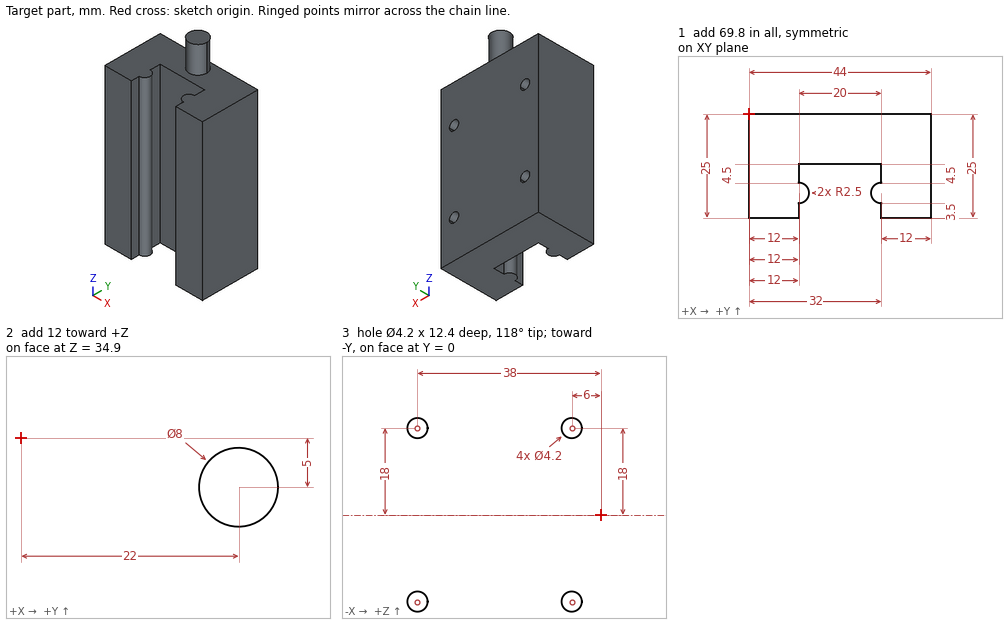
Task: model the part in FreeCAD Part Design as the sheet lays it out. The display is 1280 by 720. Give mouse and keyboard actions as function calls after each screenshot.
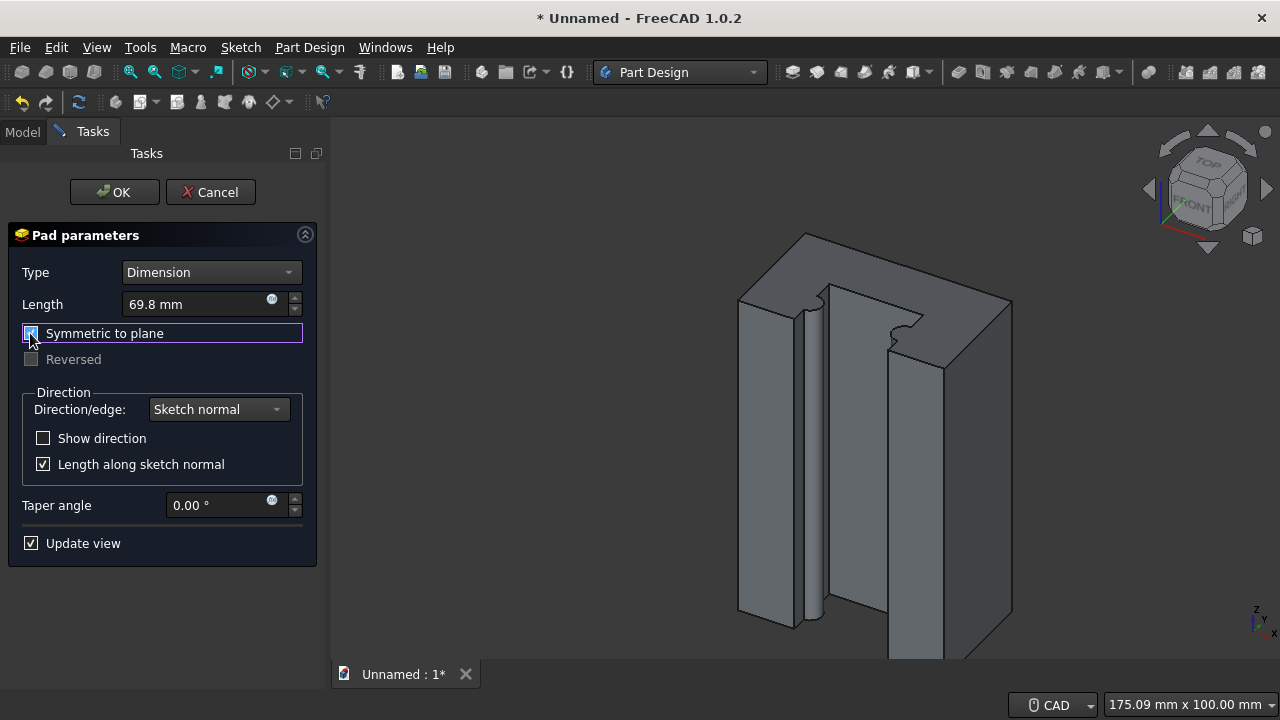
click(115, 192)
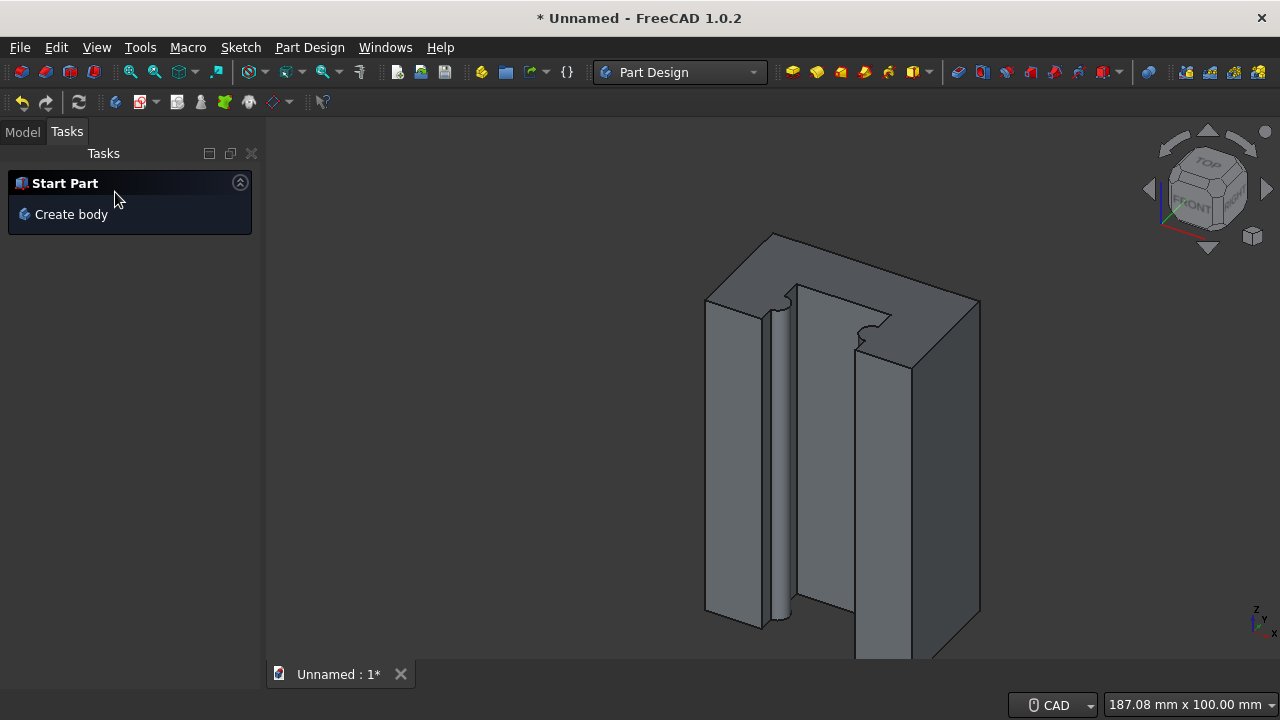
click(132, 72)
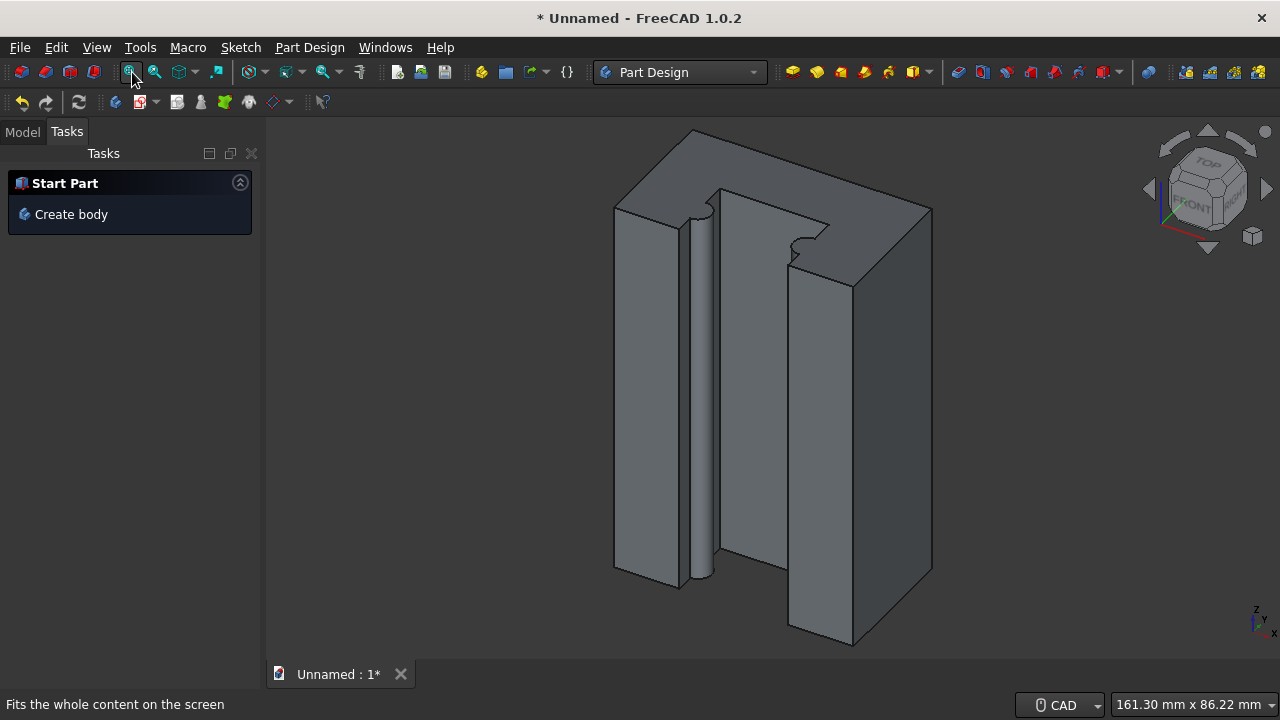
click(864, 208)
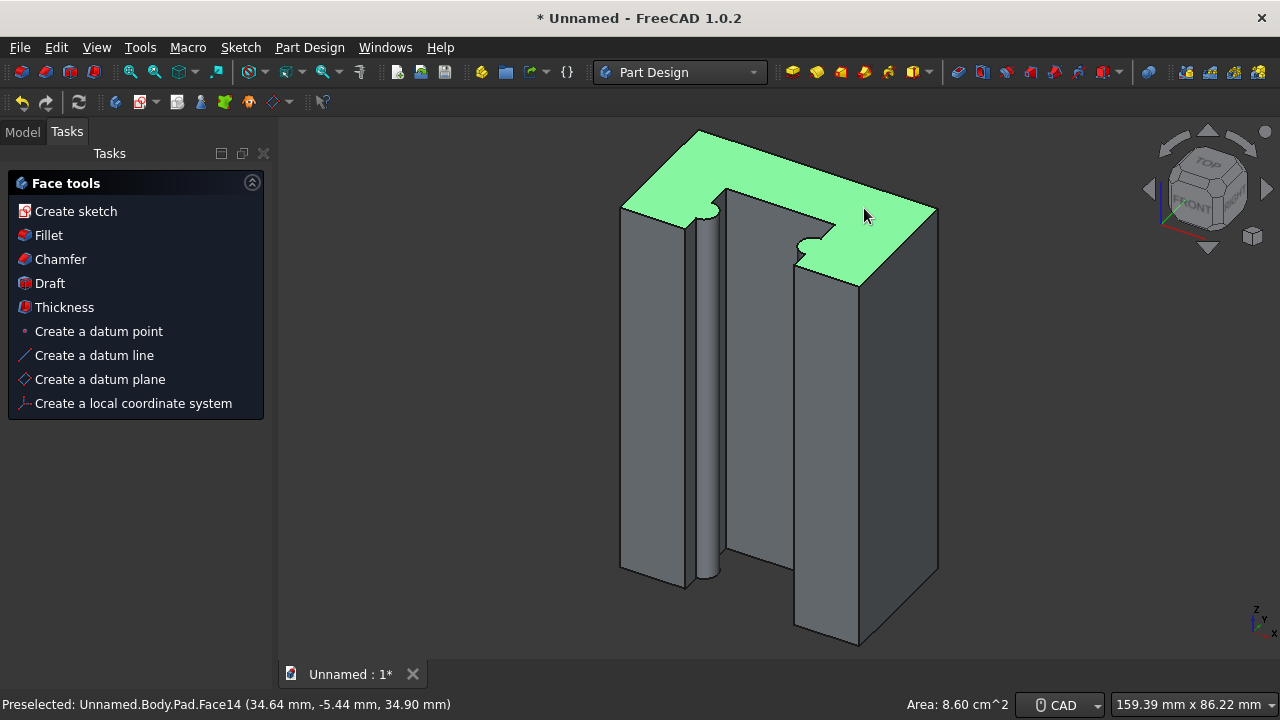
click(140, 102)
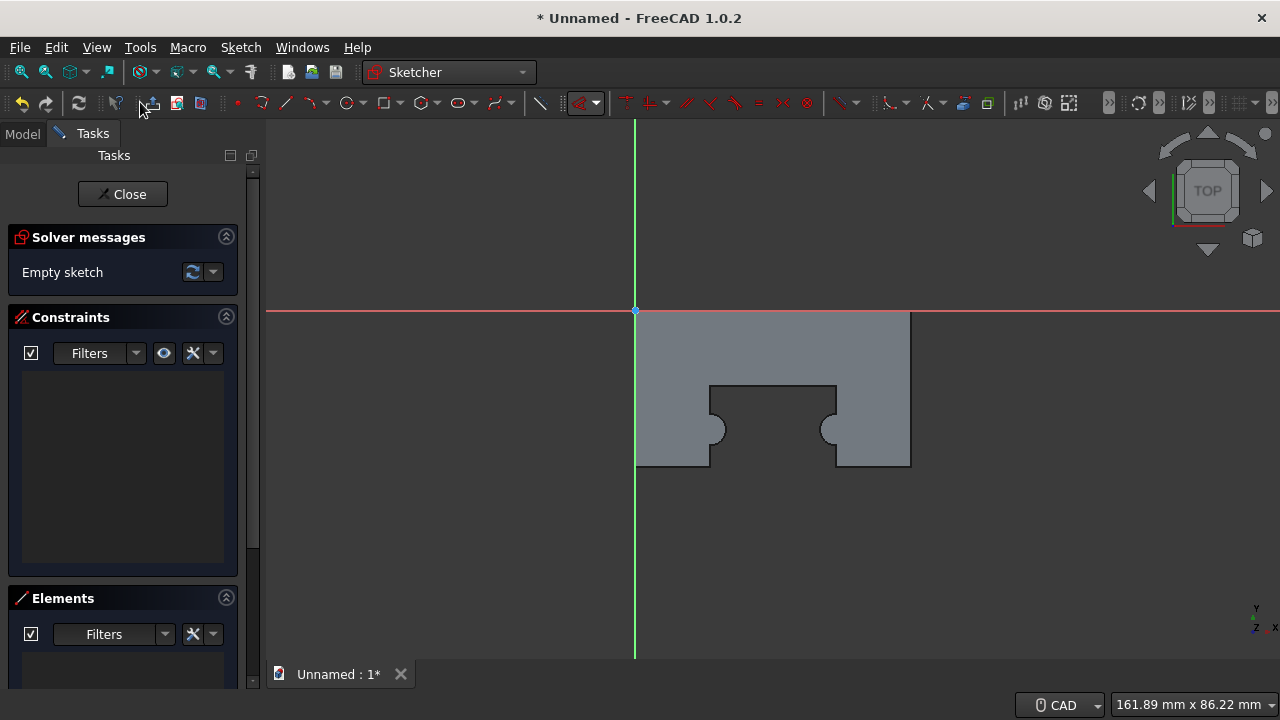
scroll(784, 335, up, 10)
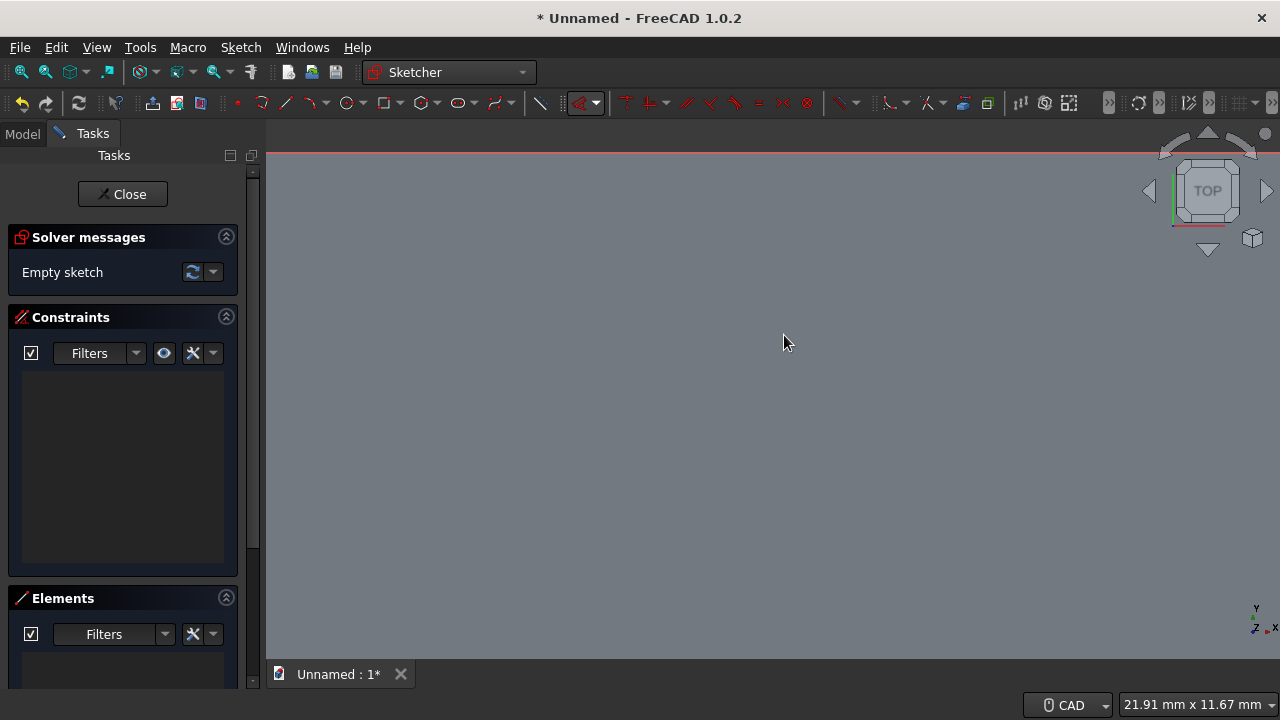
click(348, 104)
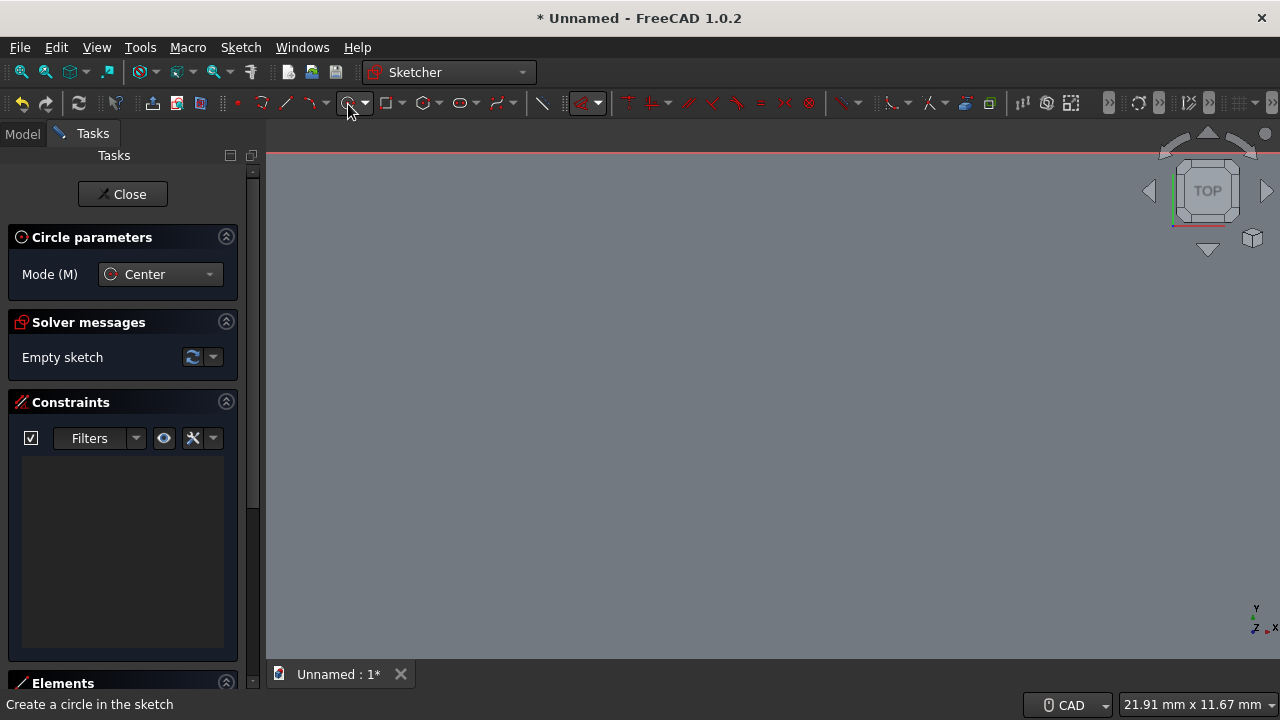
click(699, 384)
click(830, 253)
key(Escape)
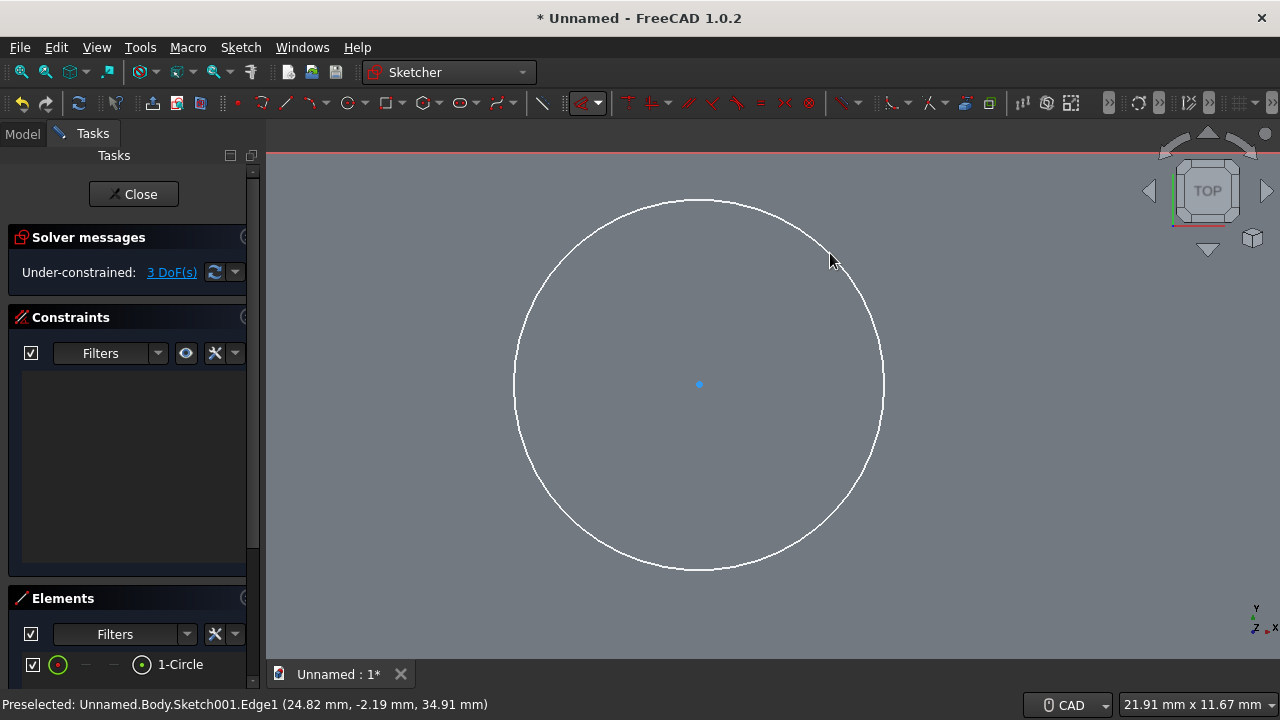
click(830, 254)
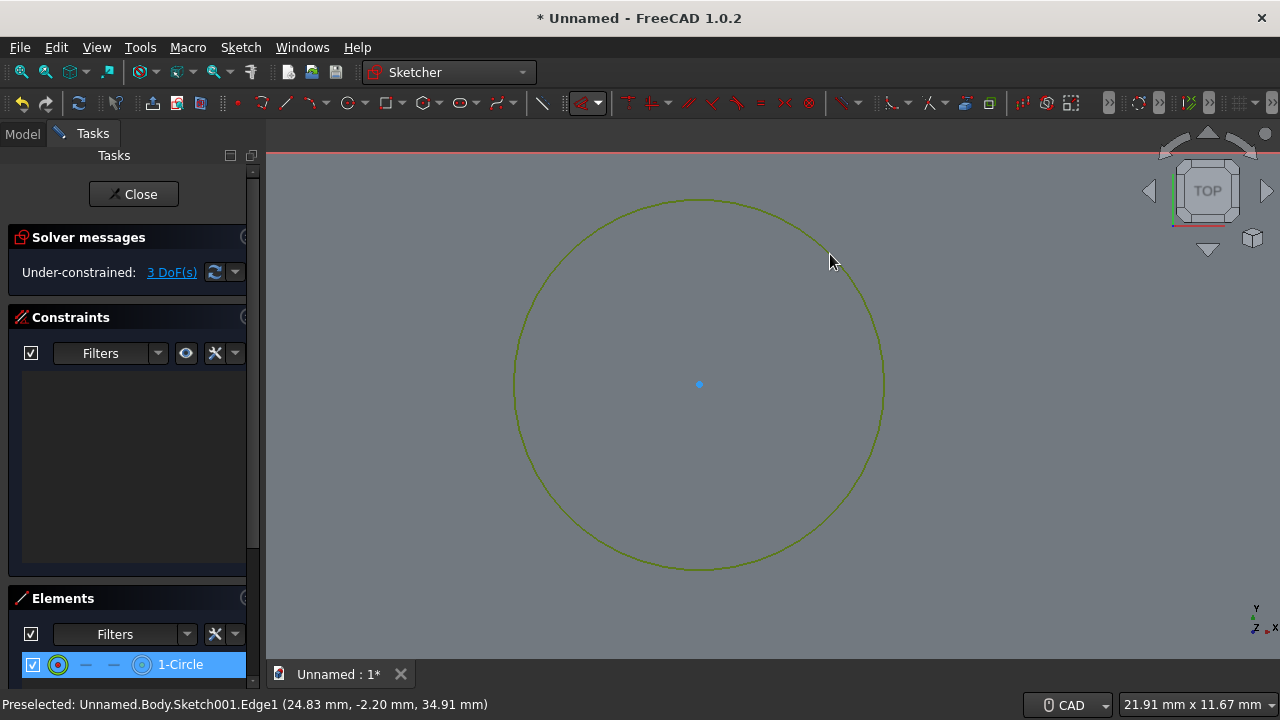
click(600, 104)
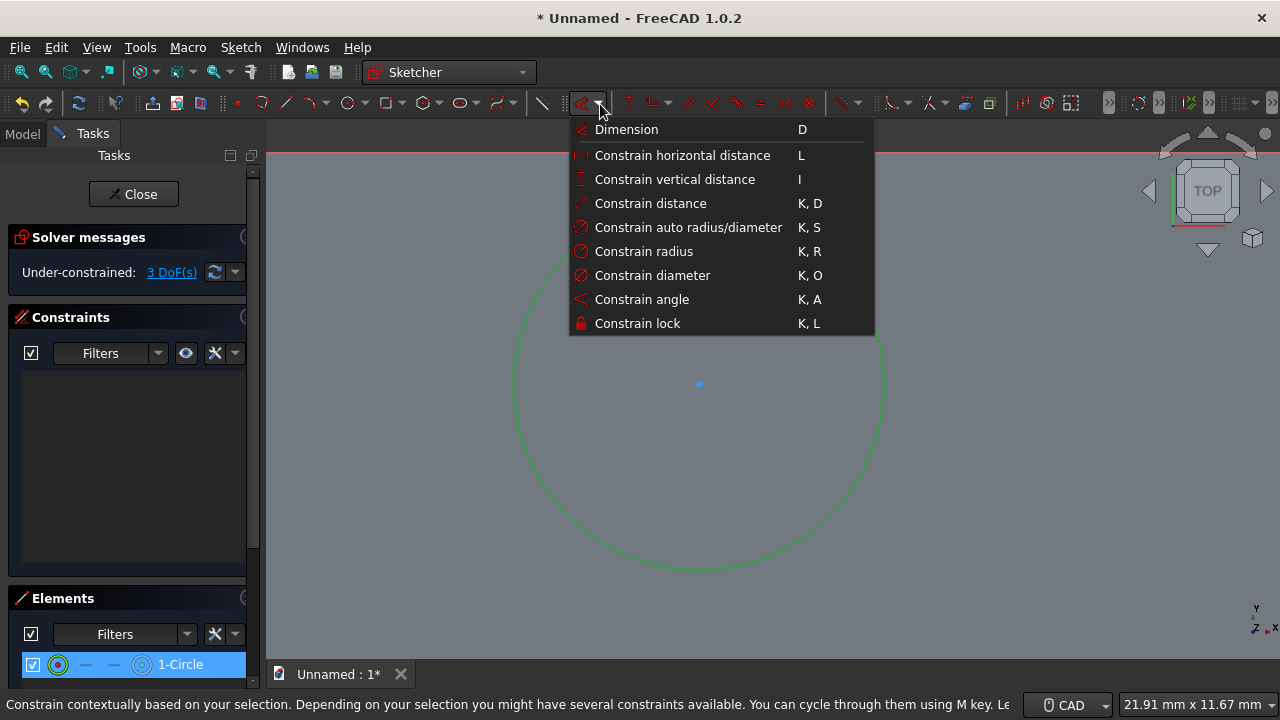
click(722, 275)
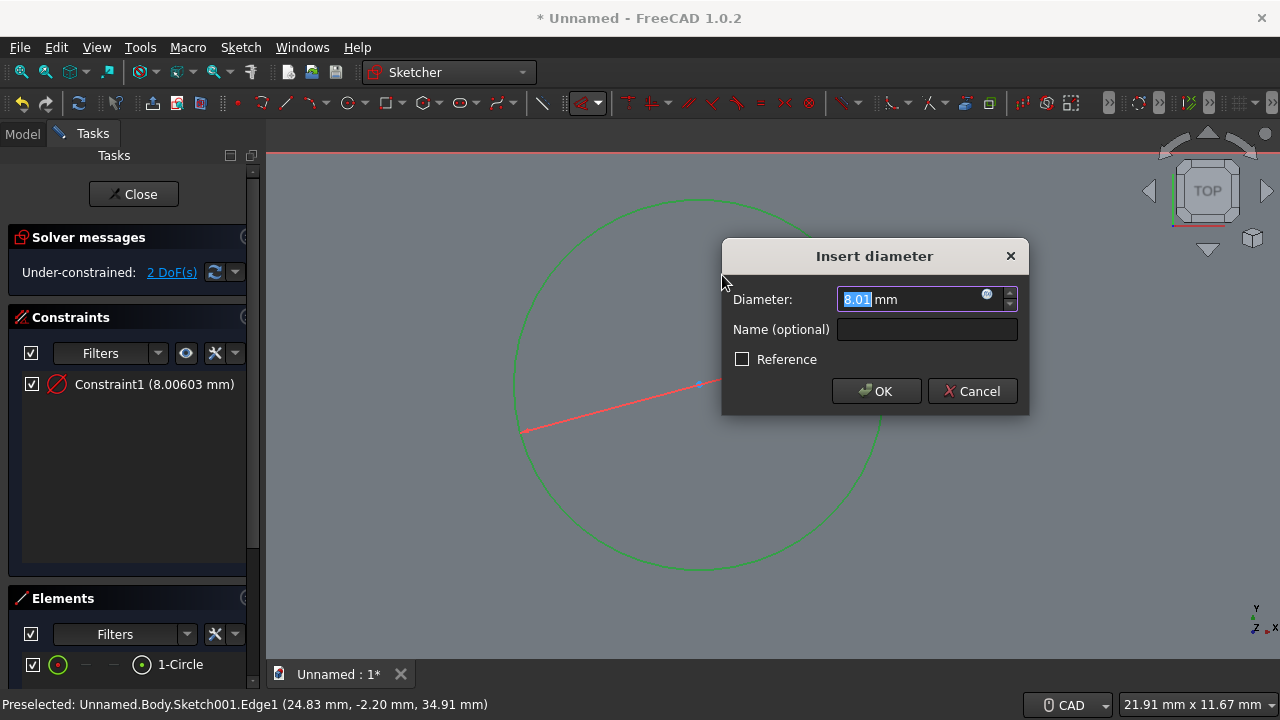
text(8)
key(Return)